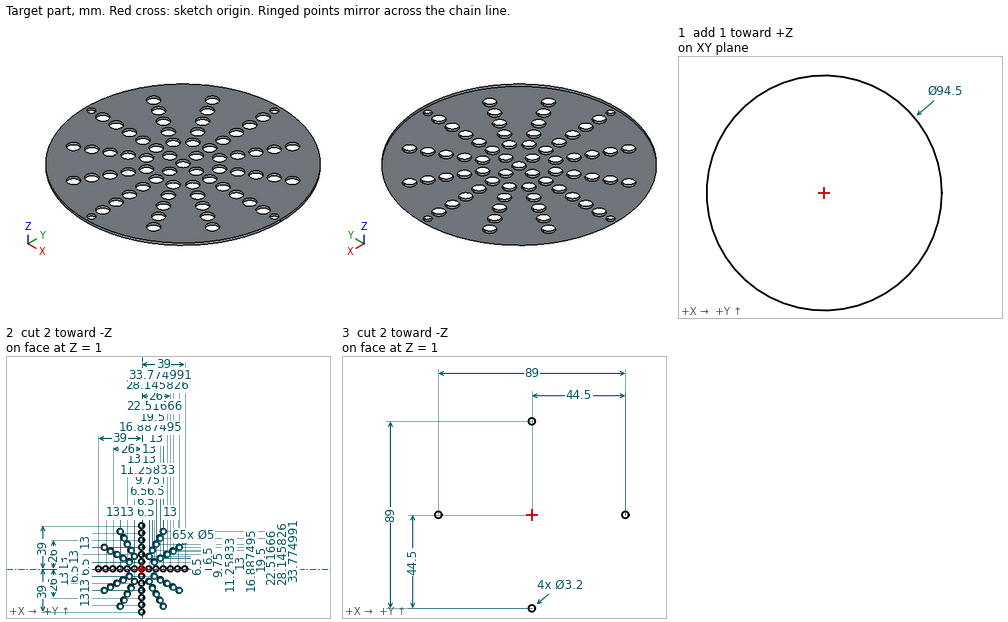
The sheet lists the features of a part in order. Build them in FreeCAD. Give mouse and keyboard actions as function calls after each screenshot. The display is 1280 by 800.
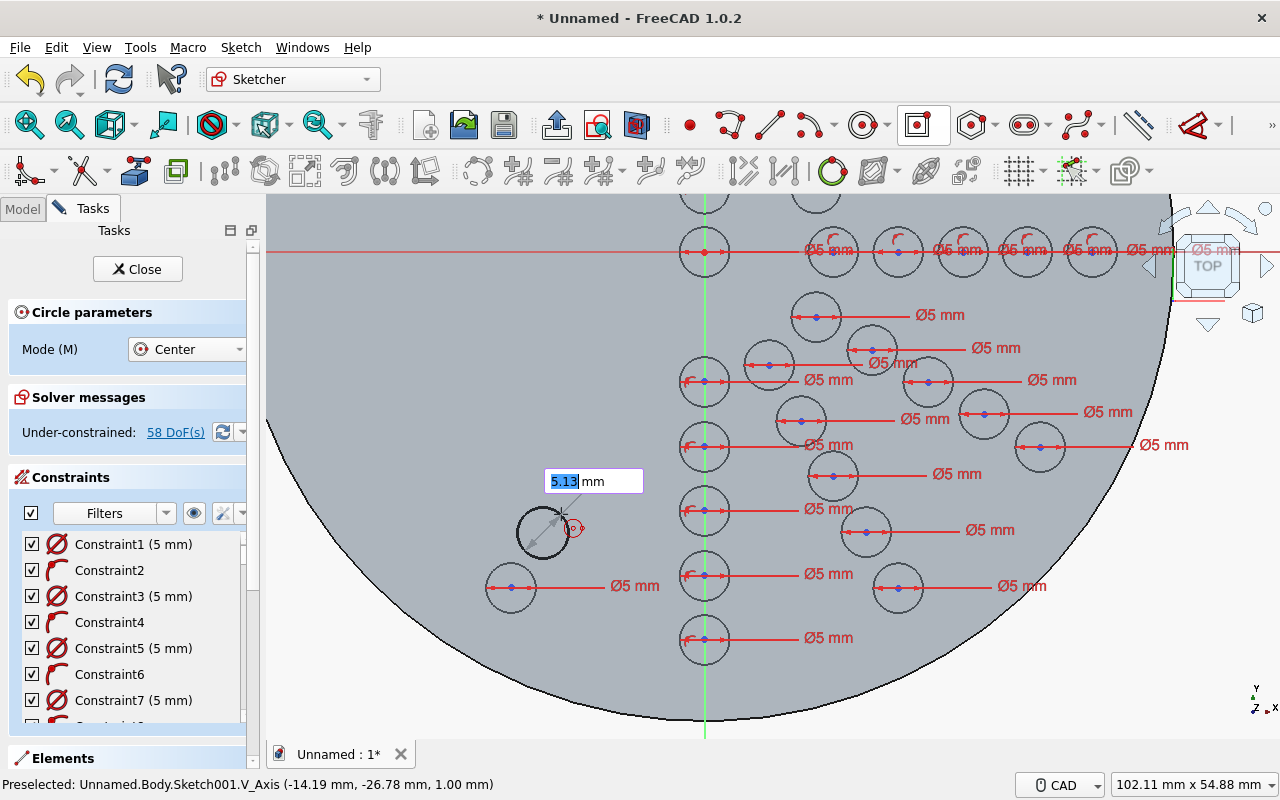
text(5)
key(Return)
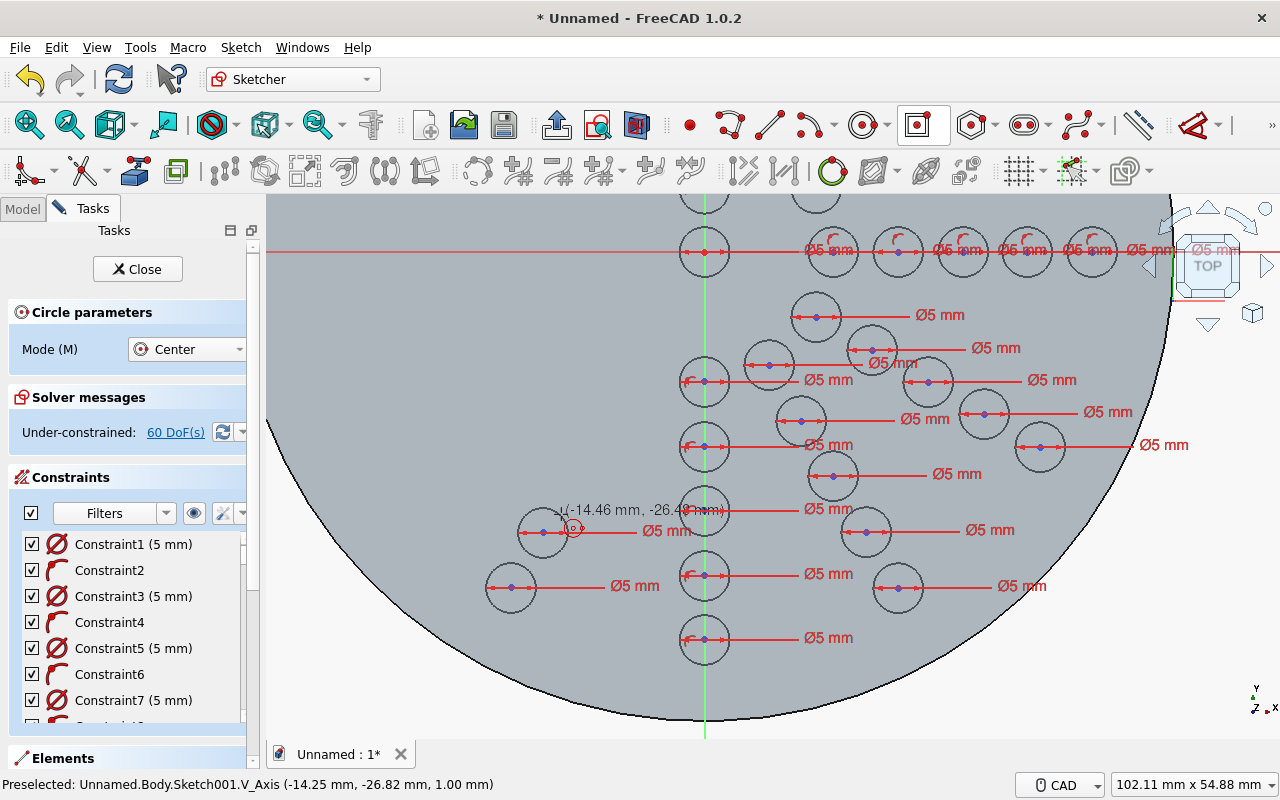
click(575, 476)
move(593, 458)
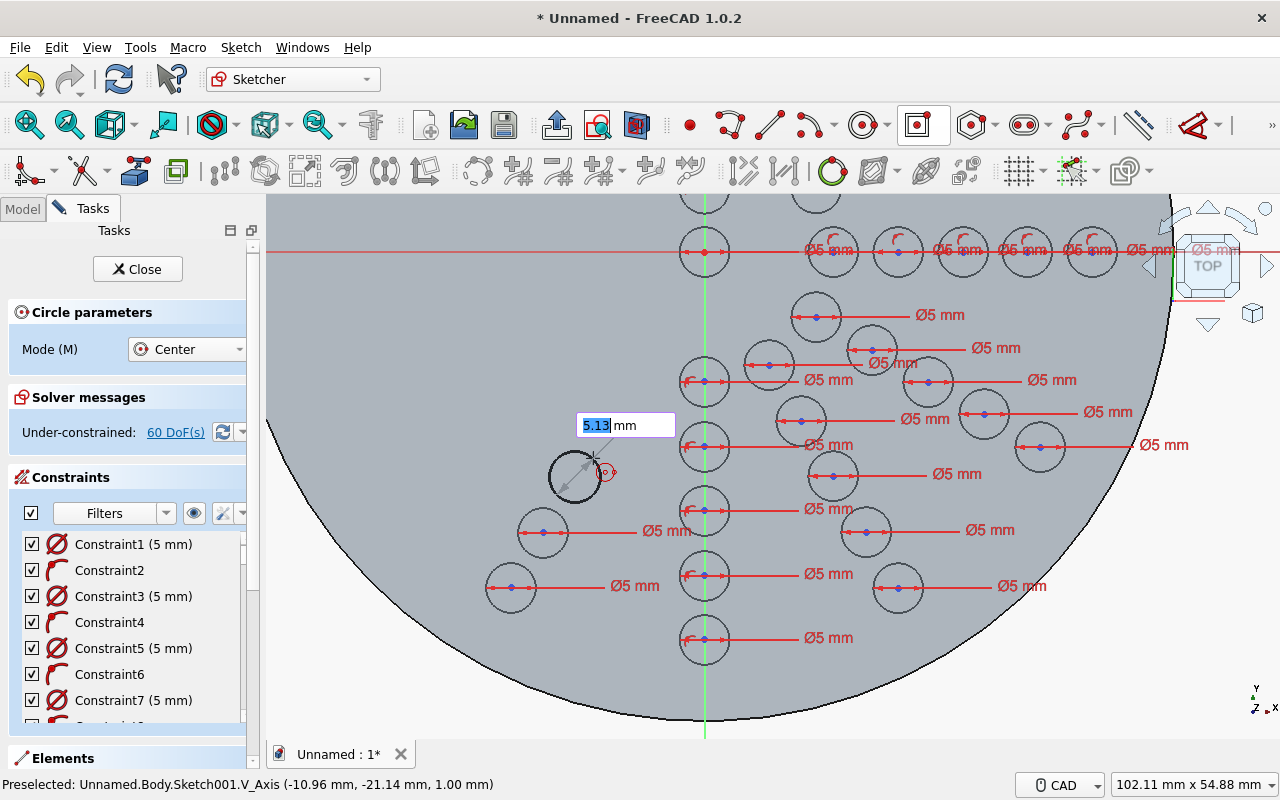
text(5)
key(Return)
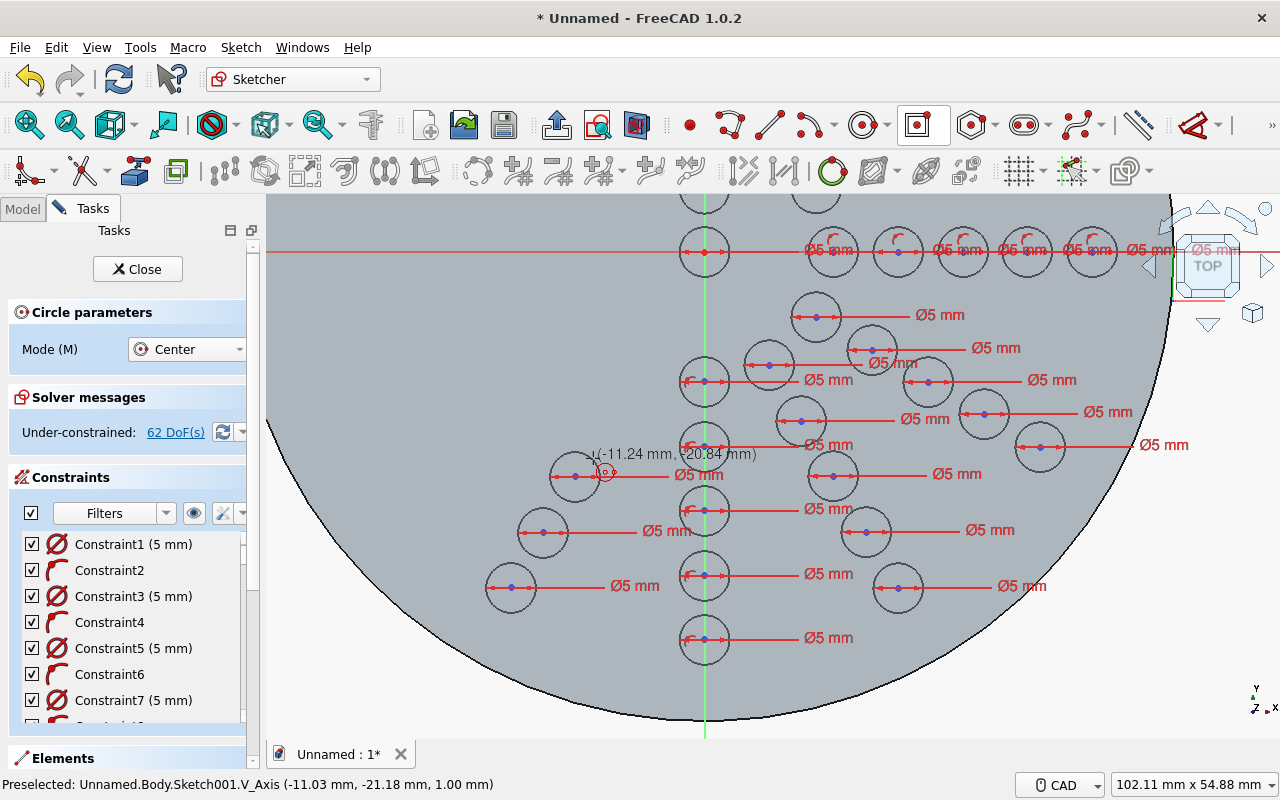
click(608, 420)
move(625, 402)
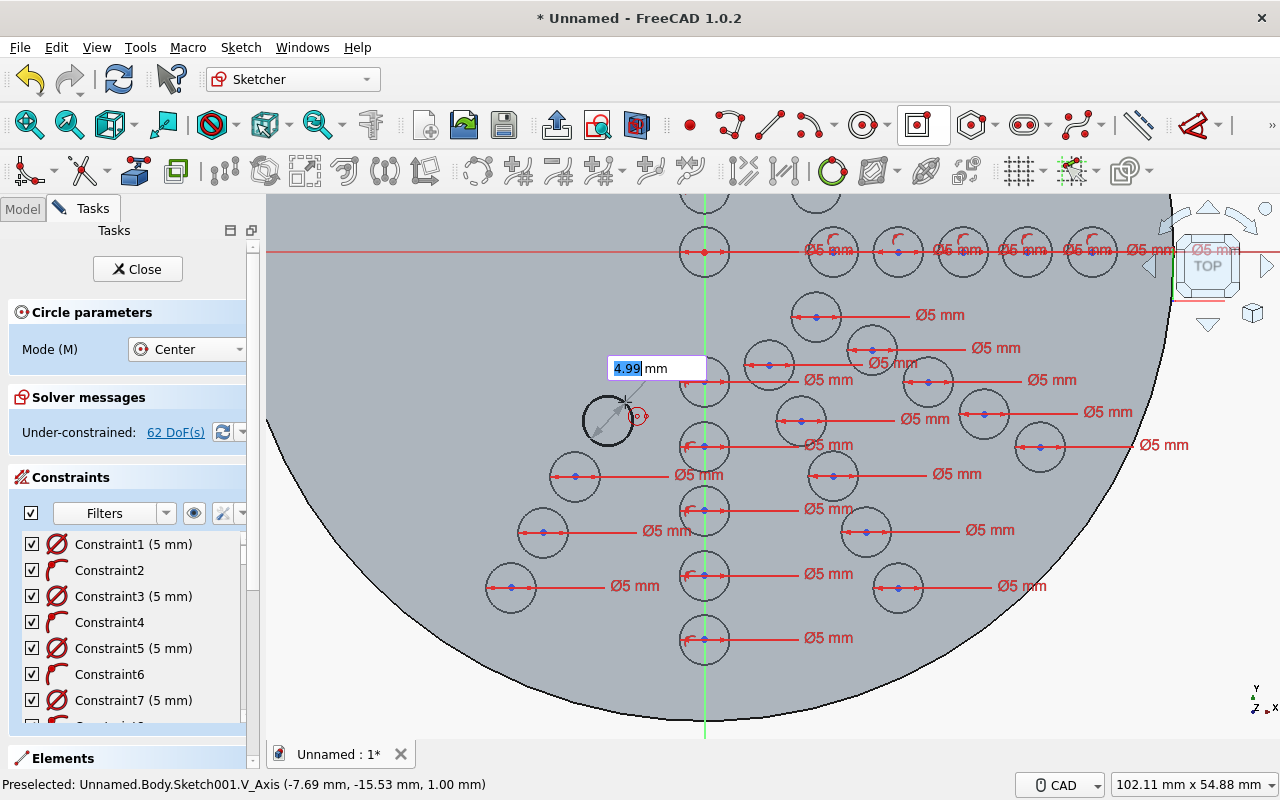
text(5)
key(Return)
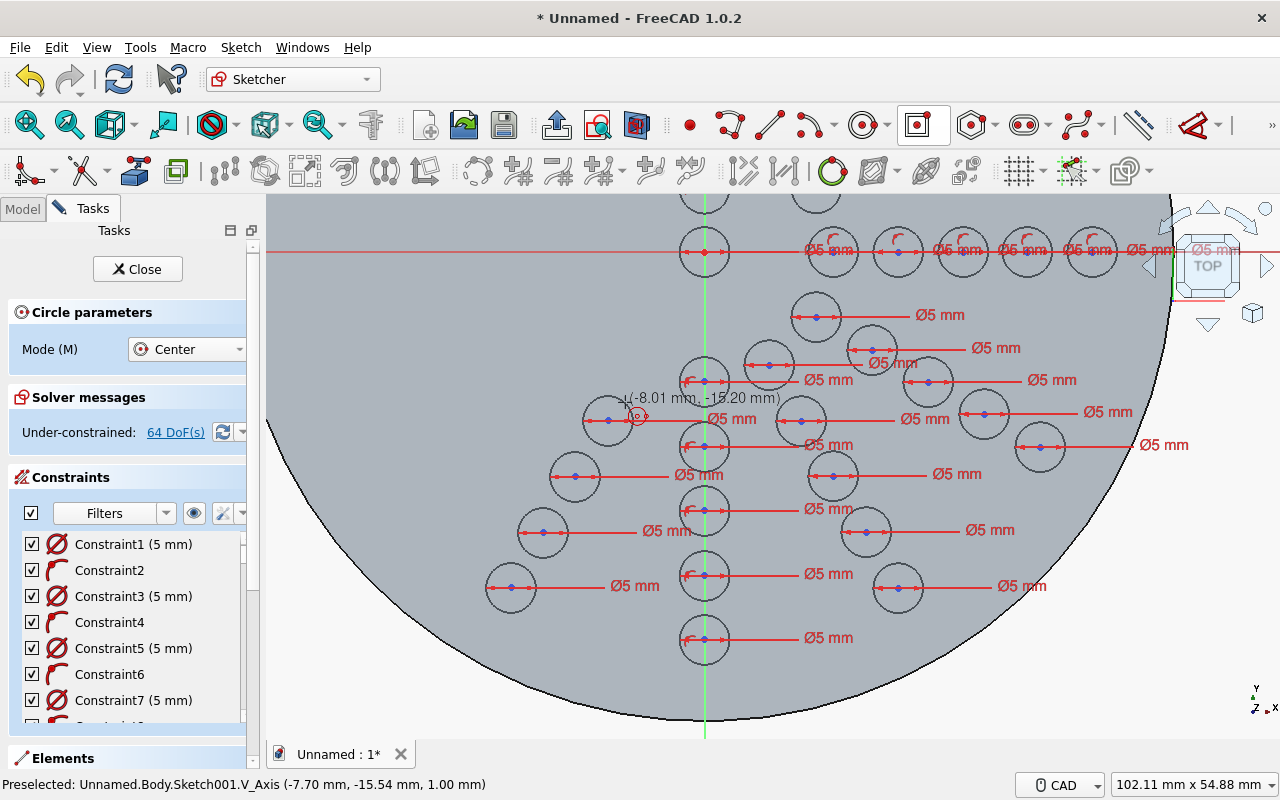
click(640, 364)
move(658, 346)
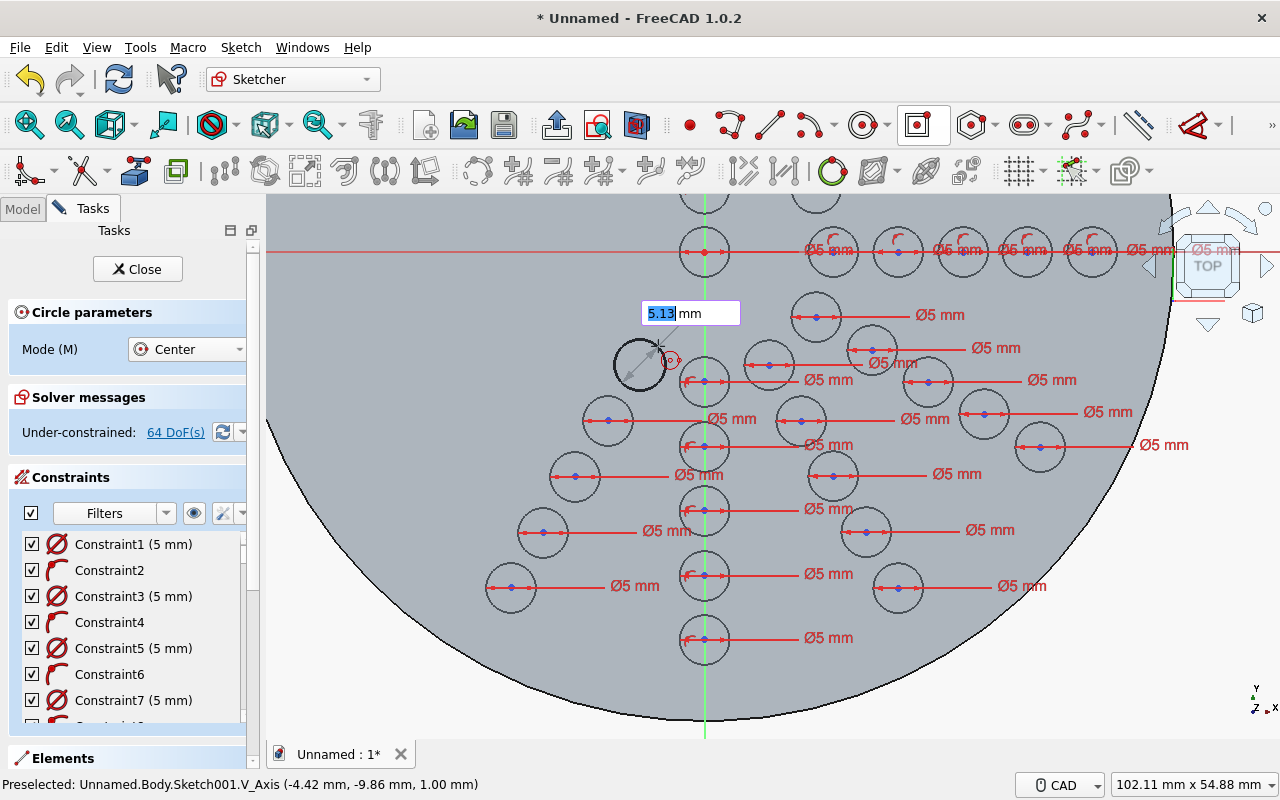
text(5)
key(Return)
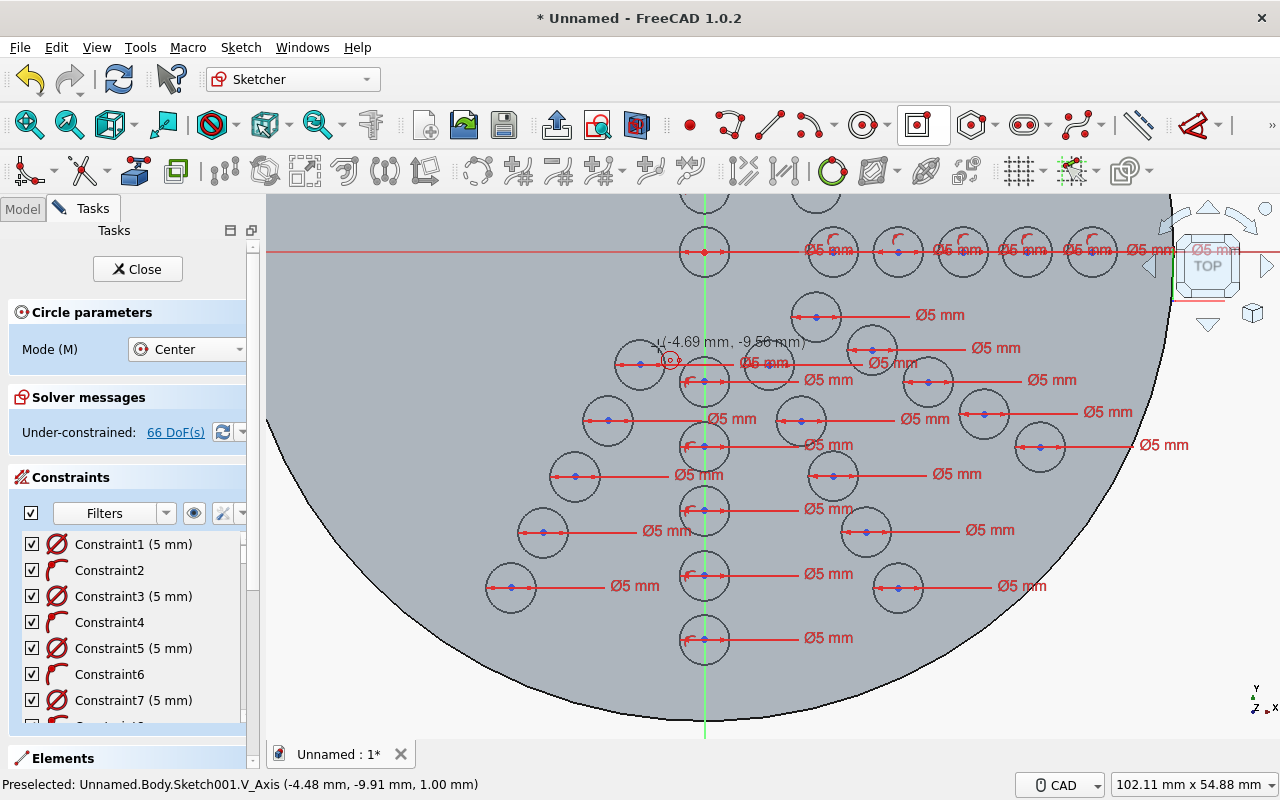
click(369, 446)
move(387, 428)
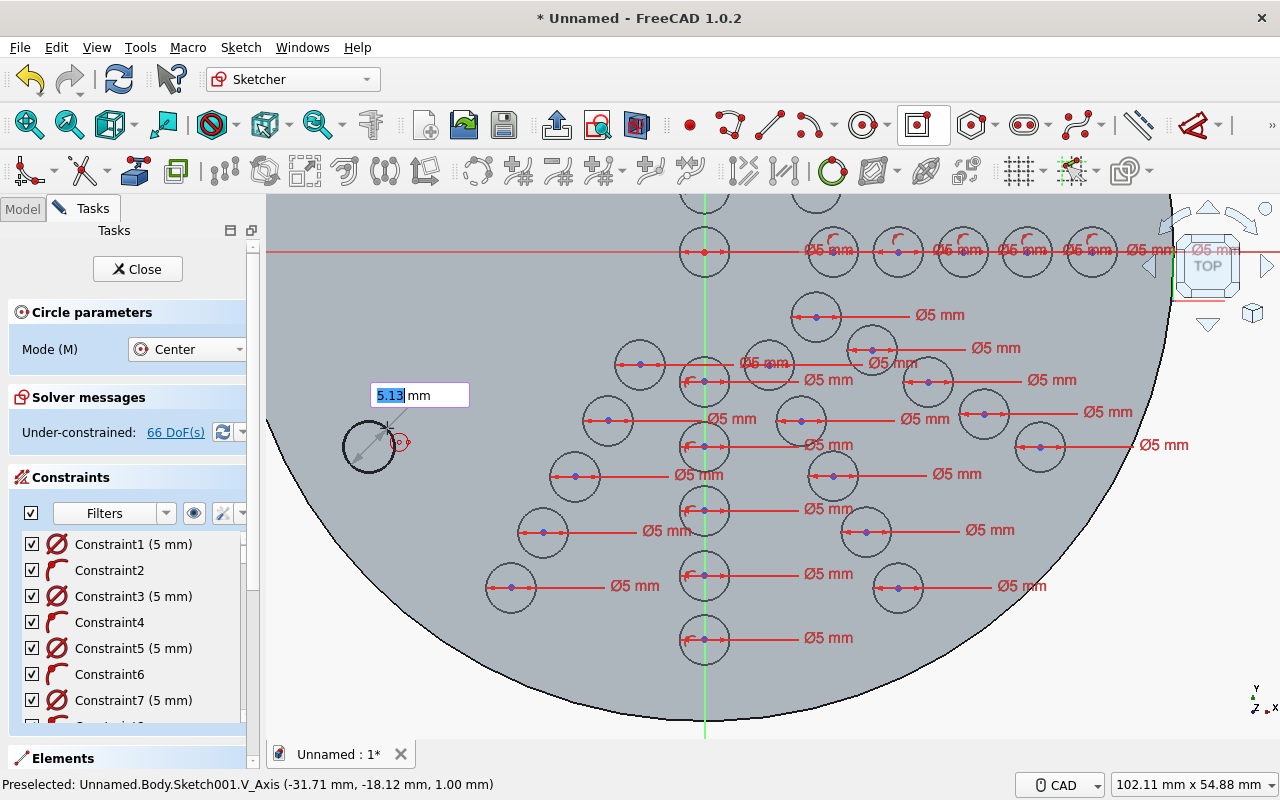
text(5)
key(Return)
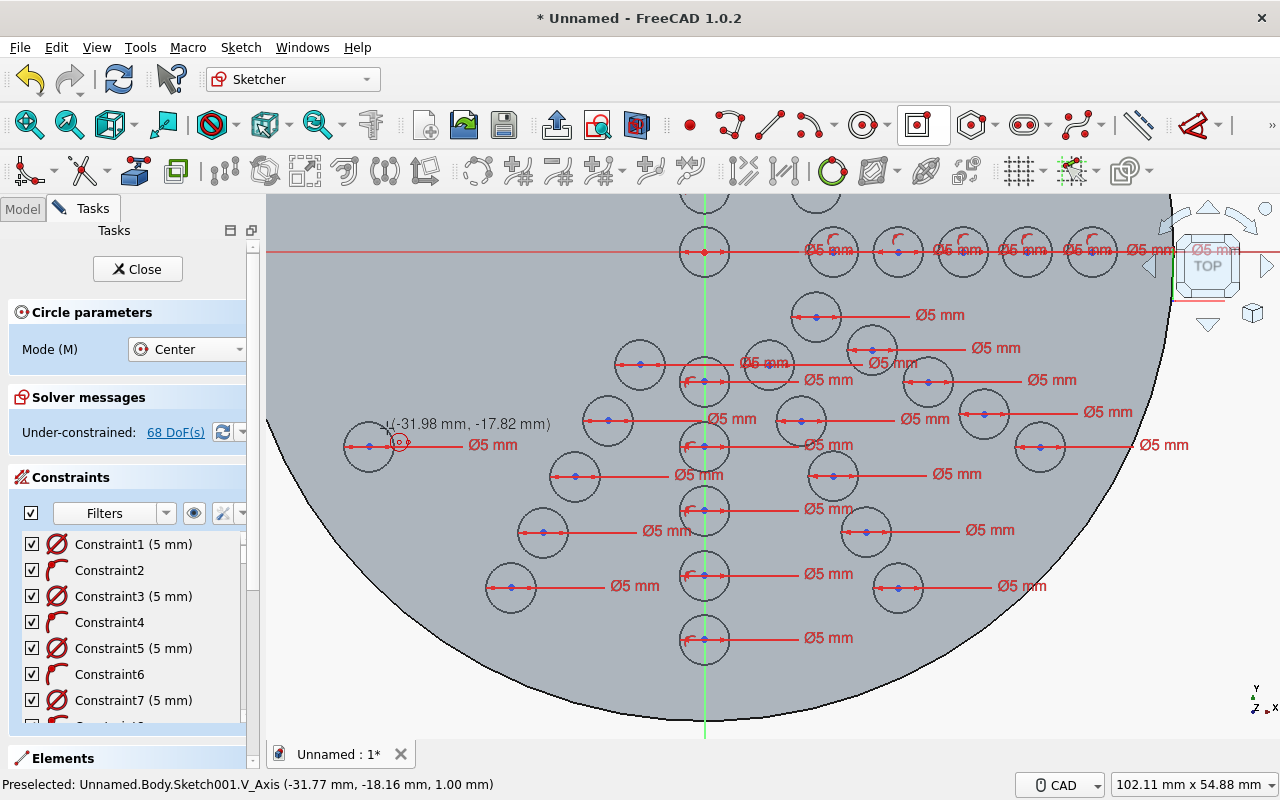
click(425, 413)
move(443, 396)